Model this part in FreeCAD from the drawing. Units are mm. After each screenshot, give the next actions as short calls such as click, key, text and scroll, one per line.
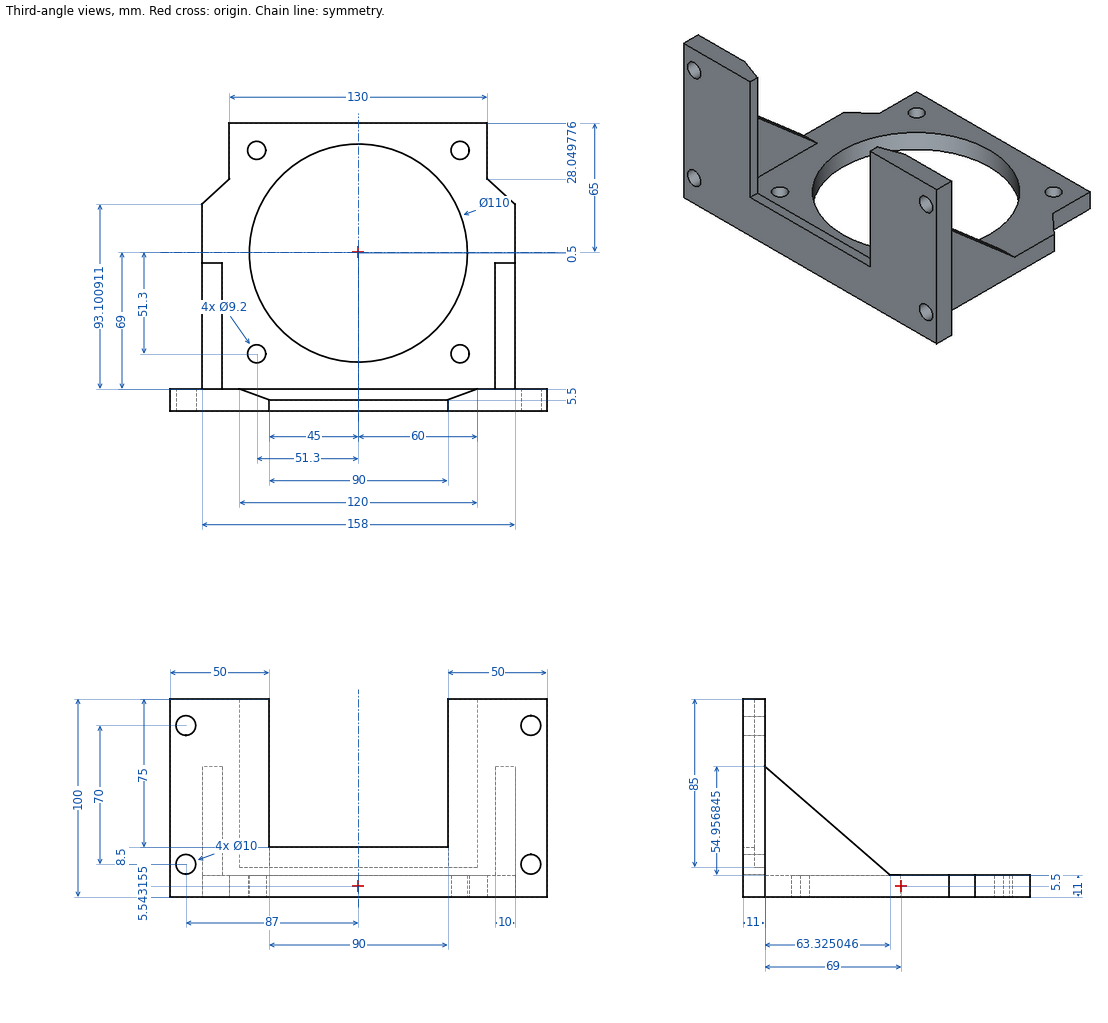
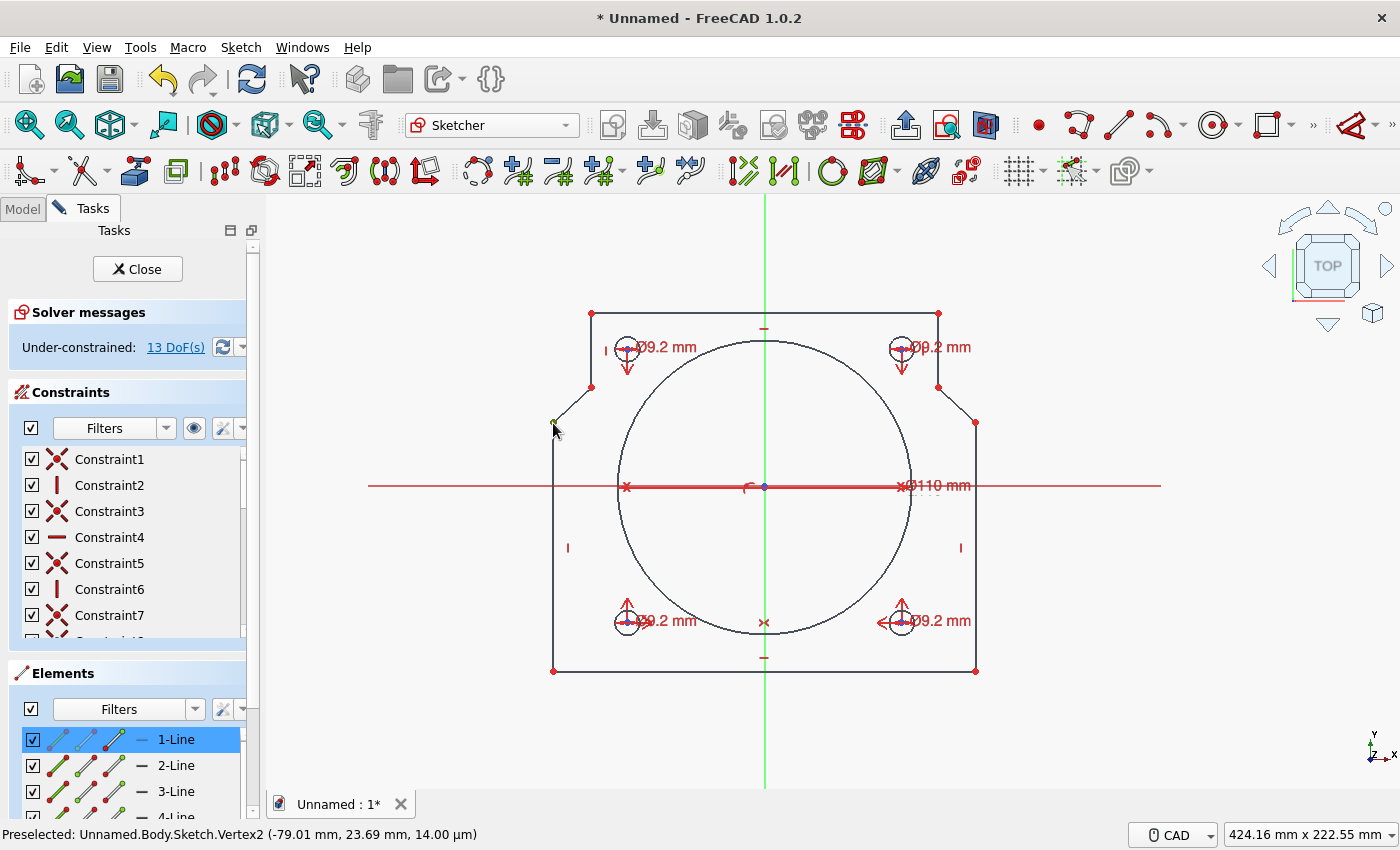
click(976, 423)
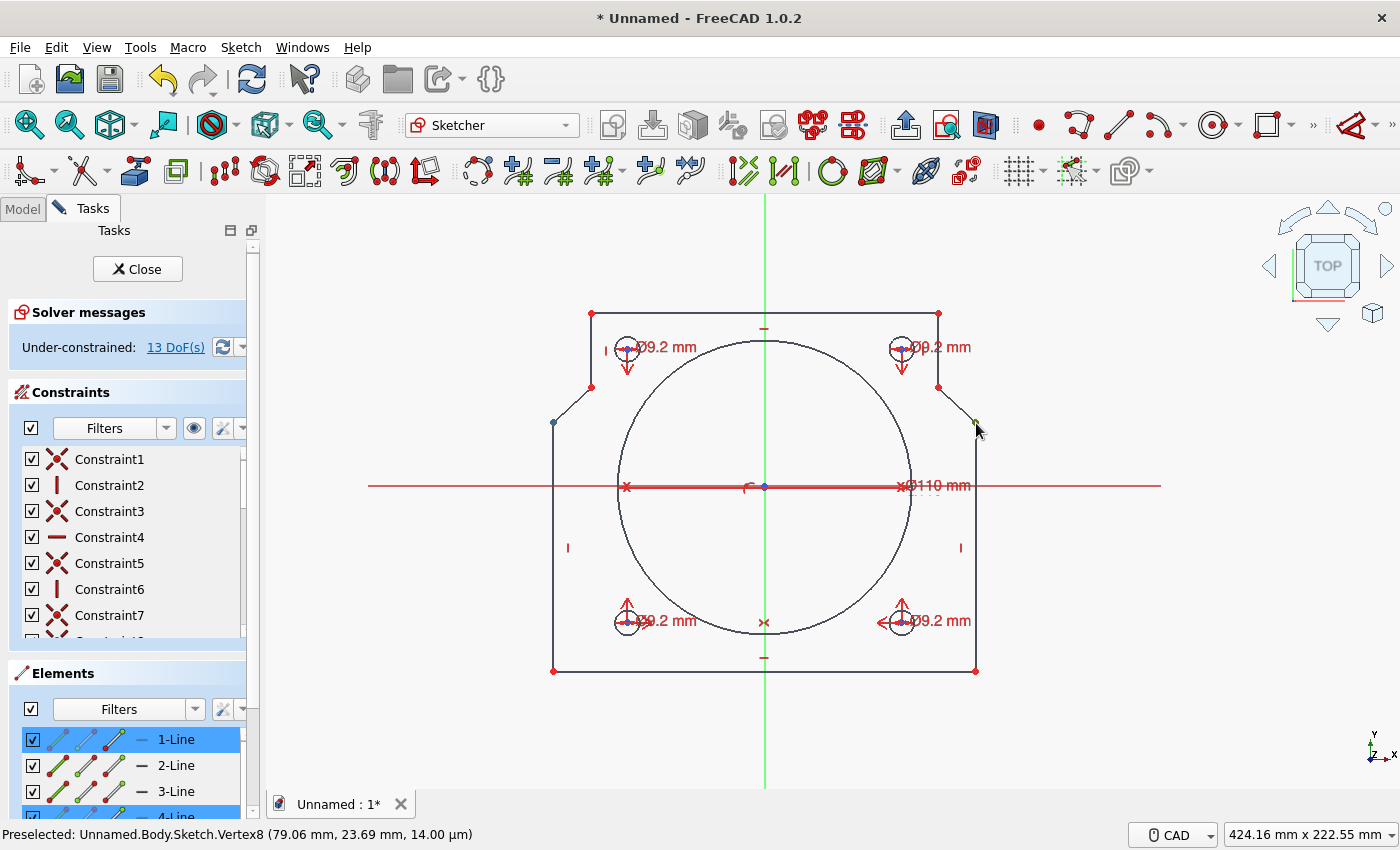
click(765, 722)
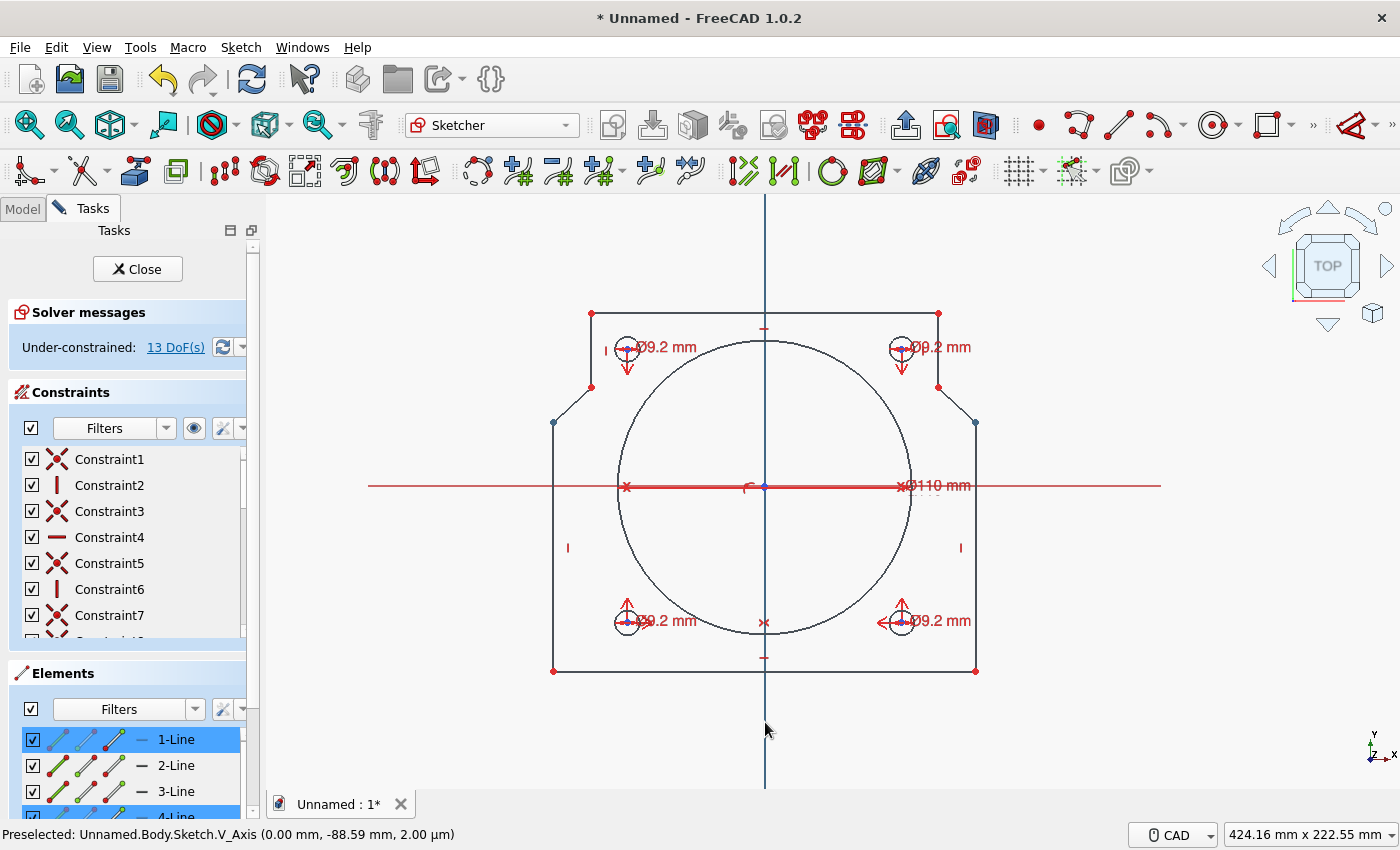
key(s)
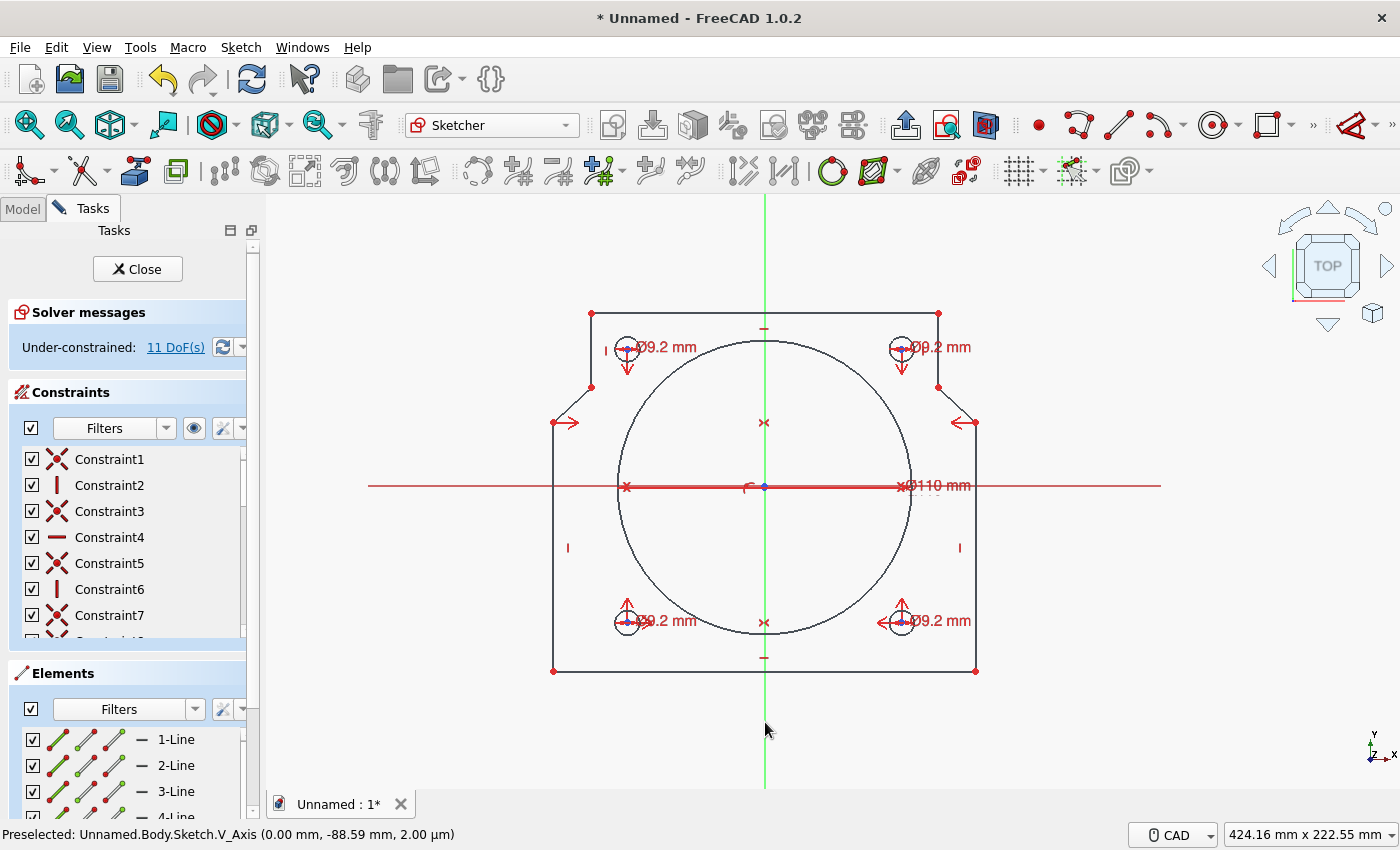
click(591, 388)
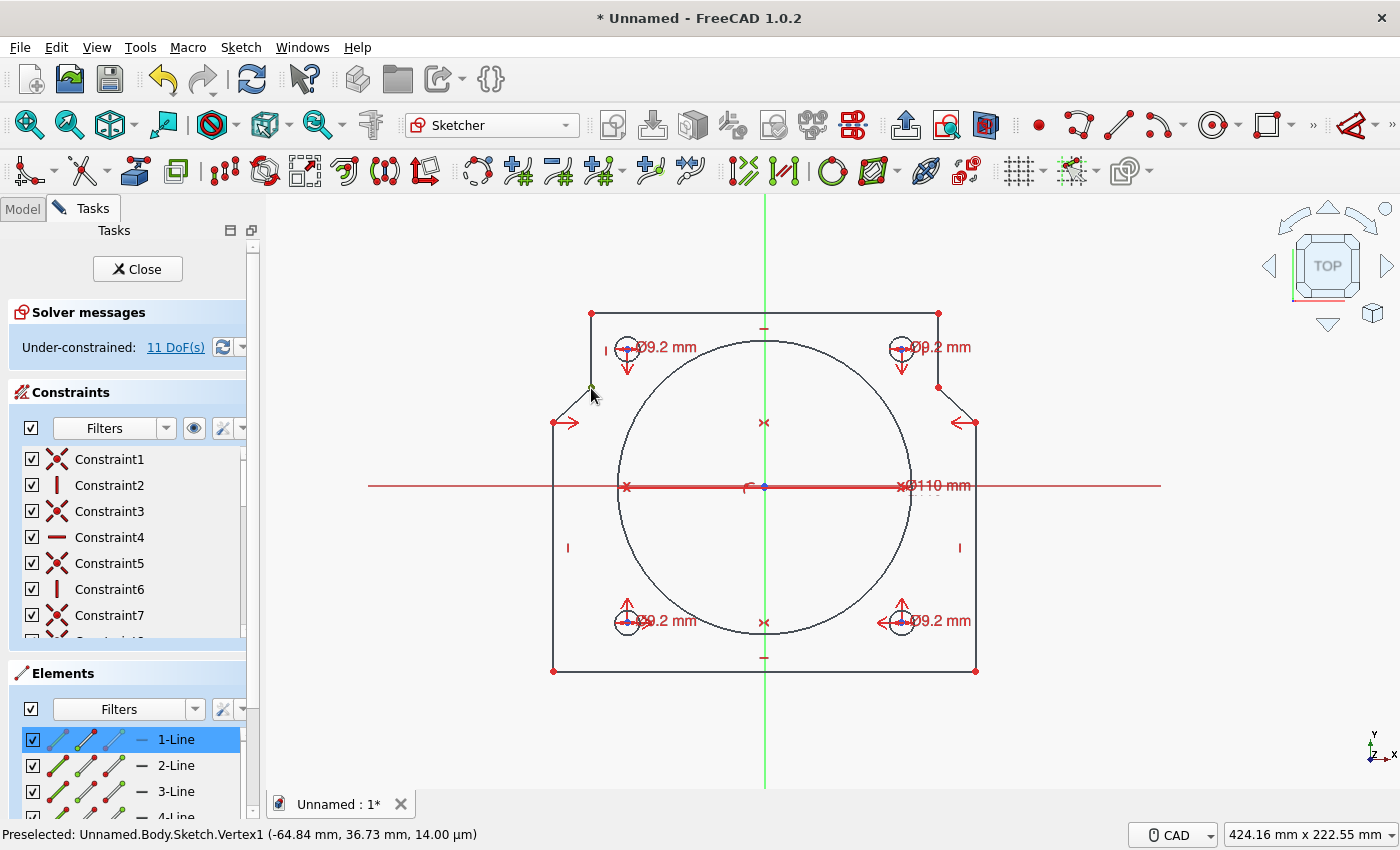
click(938, 388)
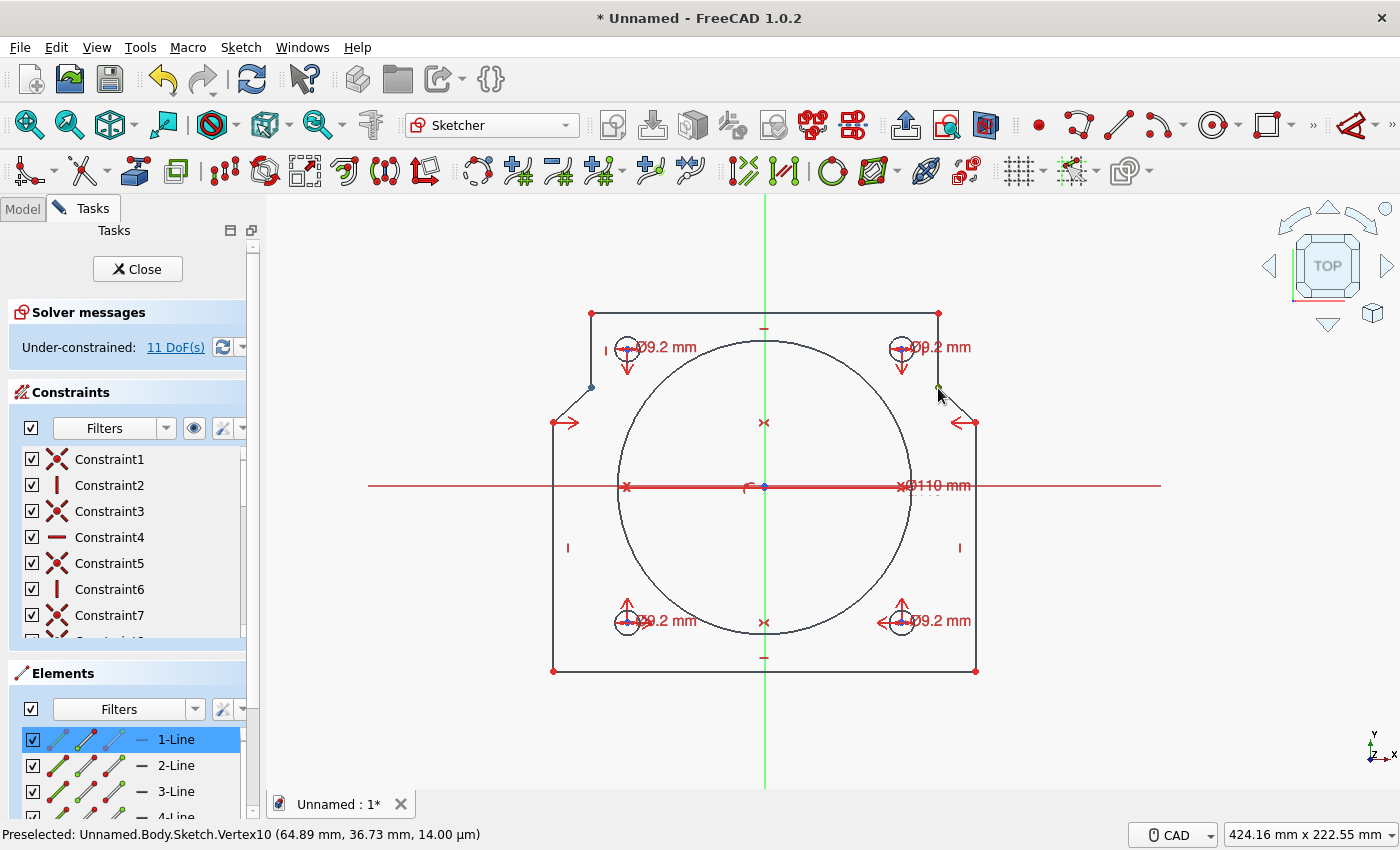
click(765, 722)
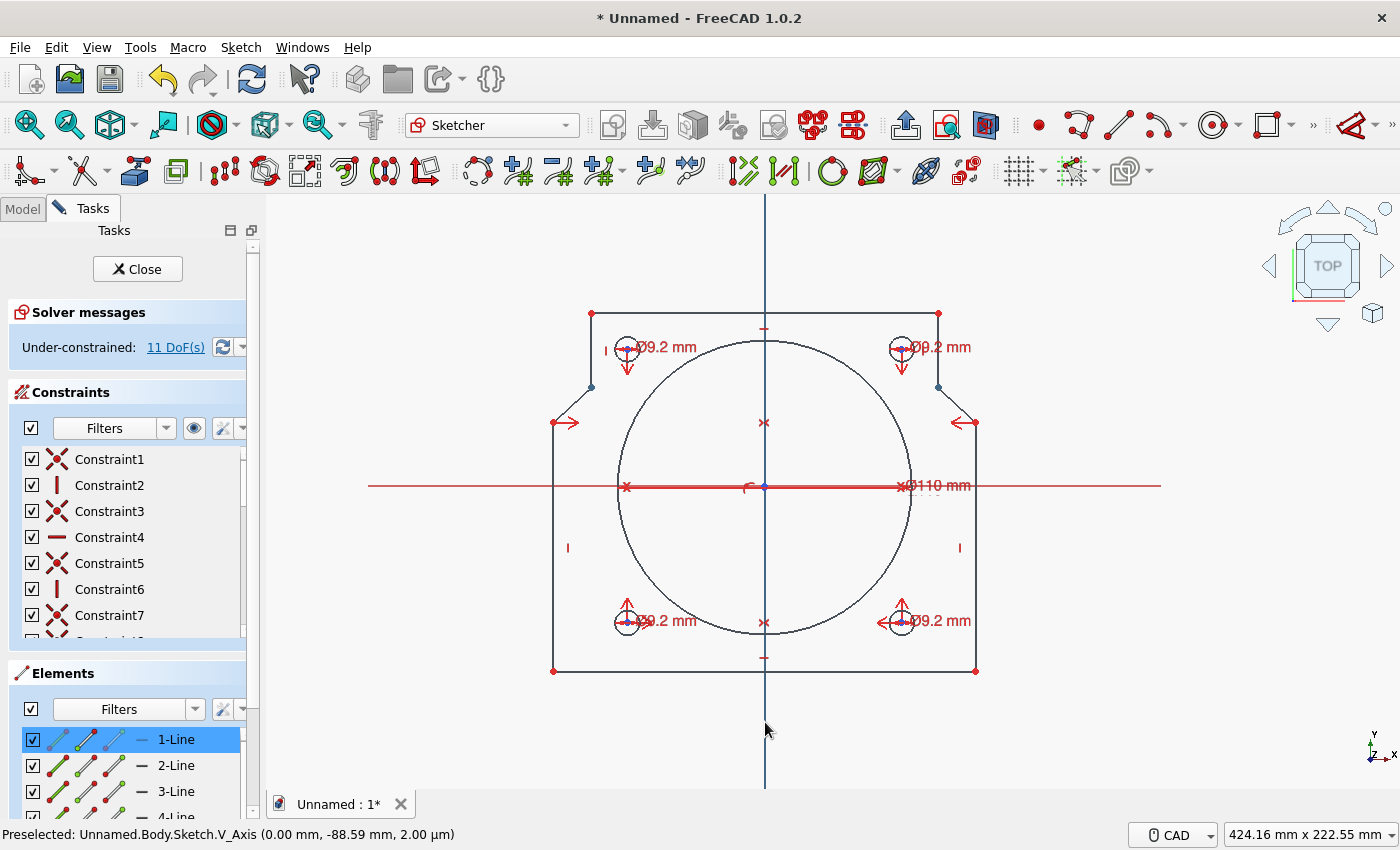
key(s)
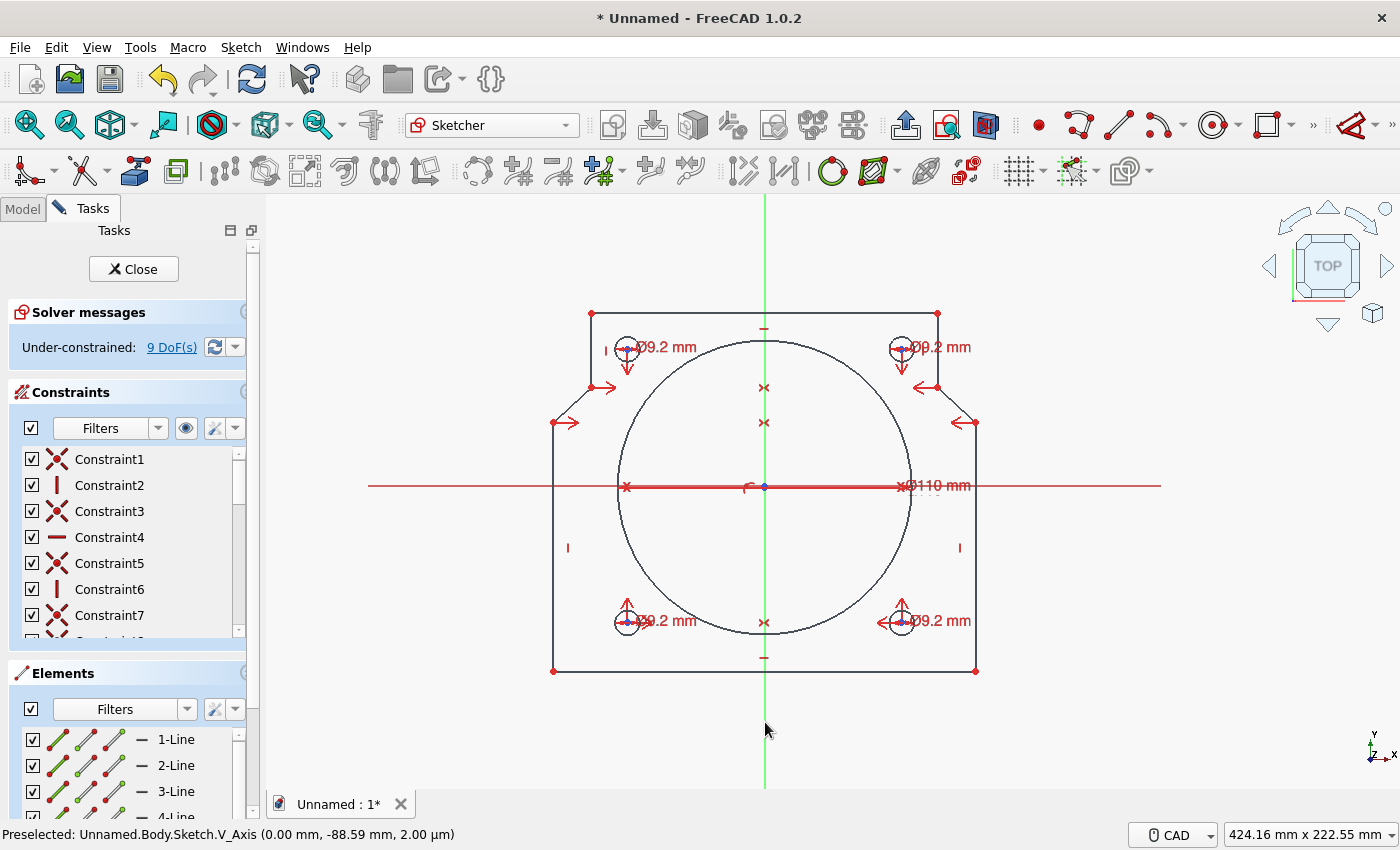
click(1352, 126)